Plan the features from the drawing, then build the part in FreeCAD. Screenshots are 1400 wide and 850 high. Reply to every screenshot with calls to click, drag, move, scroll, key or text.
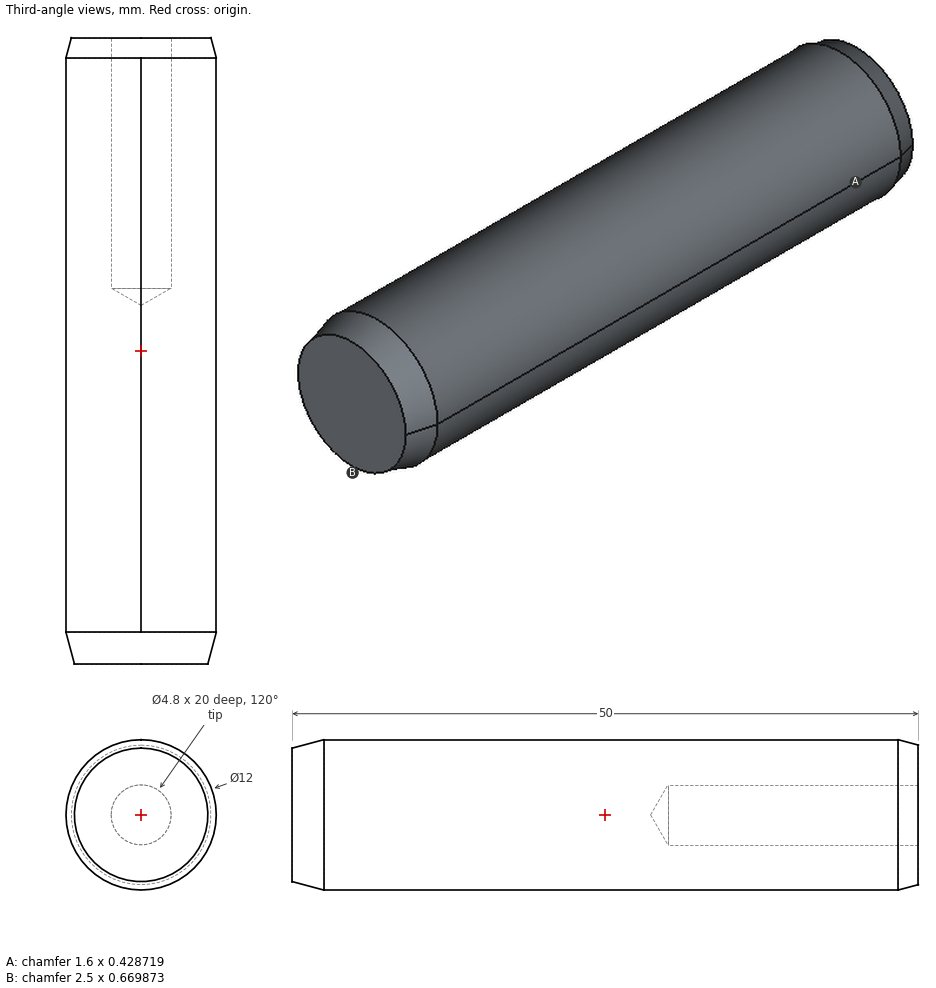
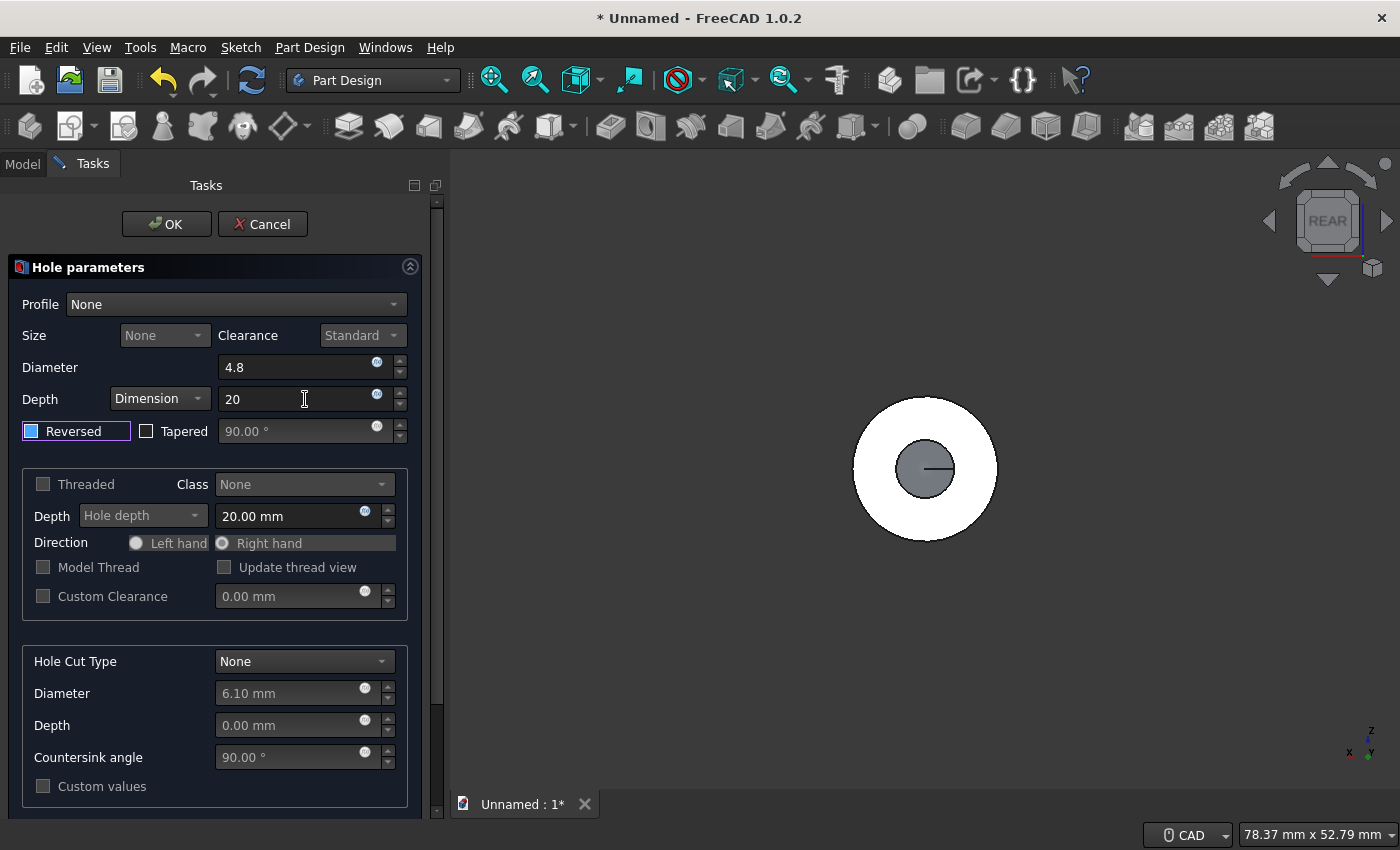
scroll(437, 506, down, 3)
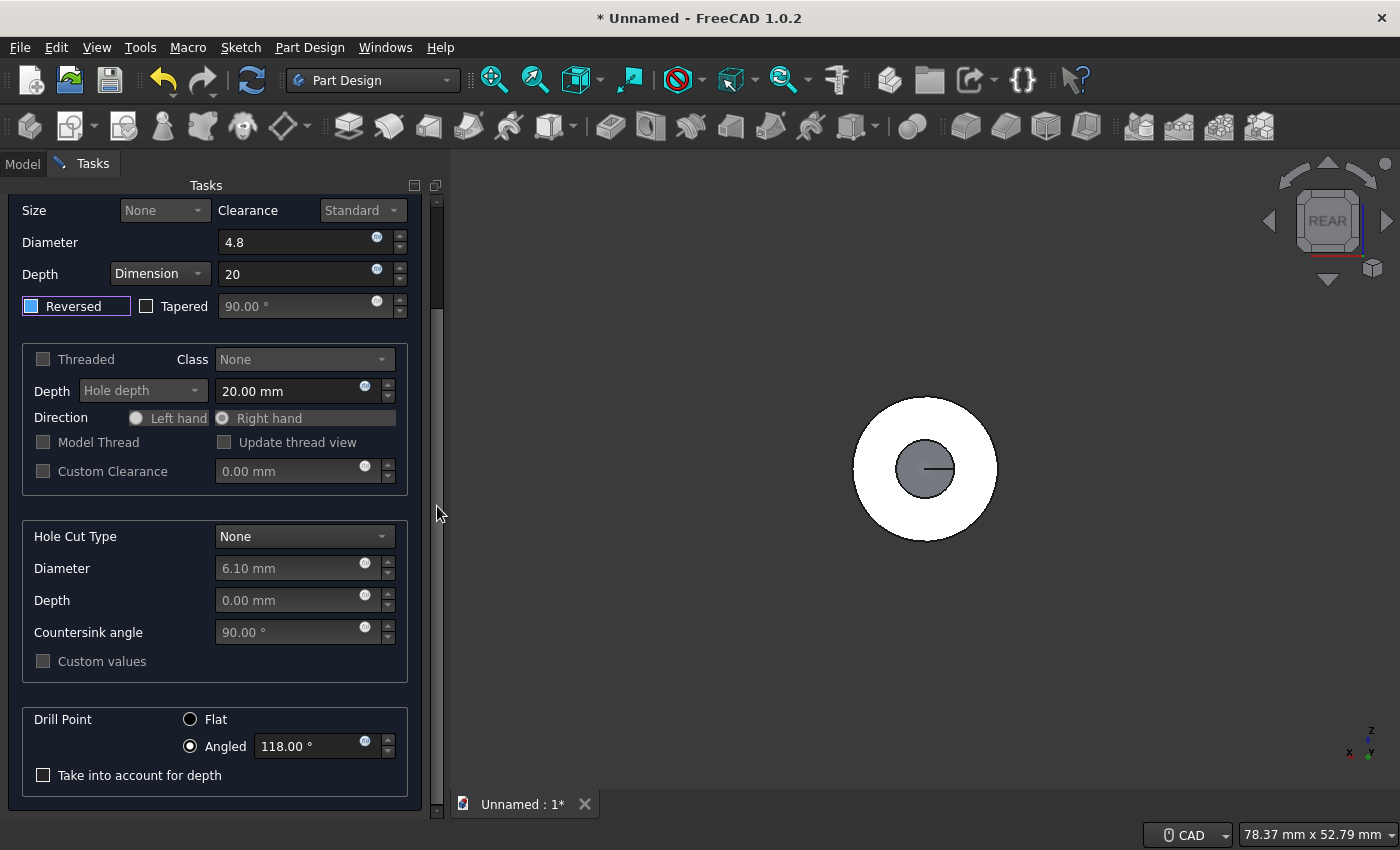
triple_click(317, 746)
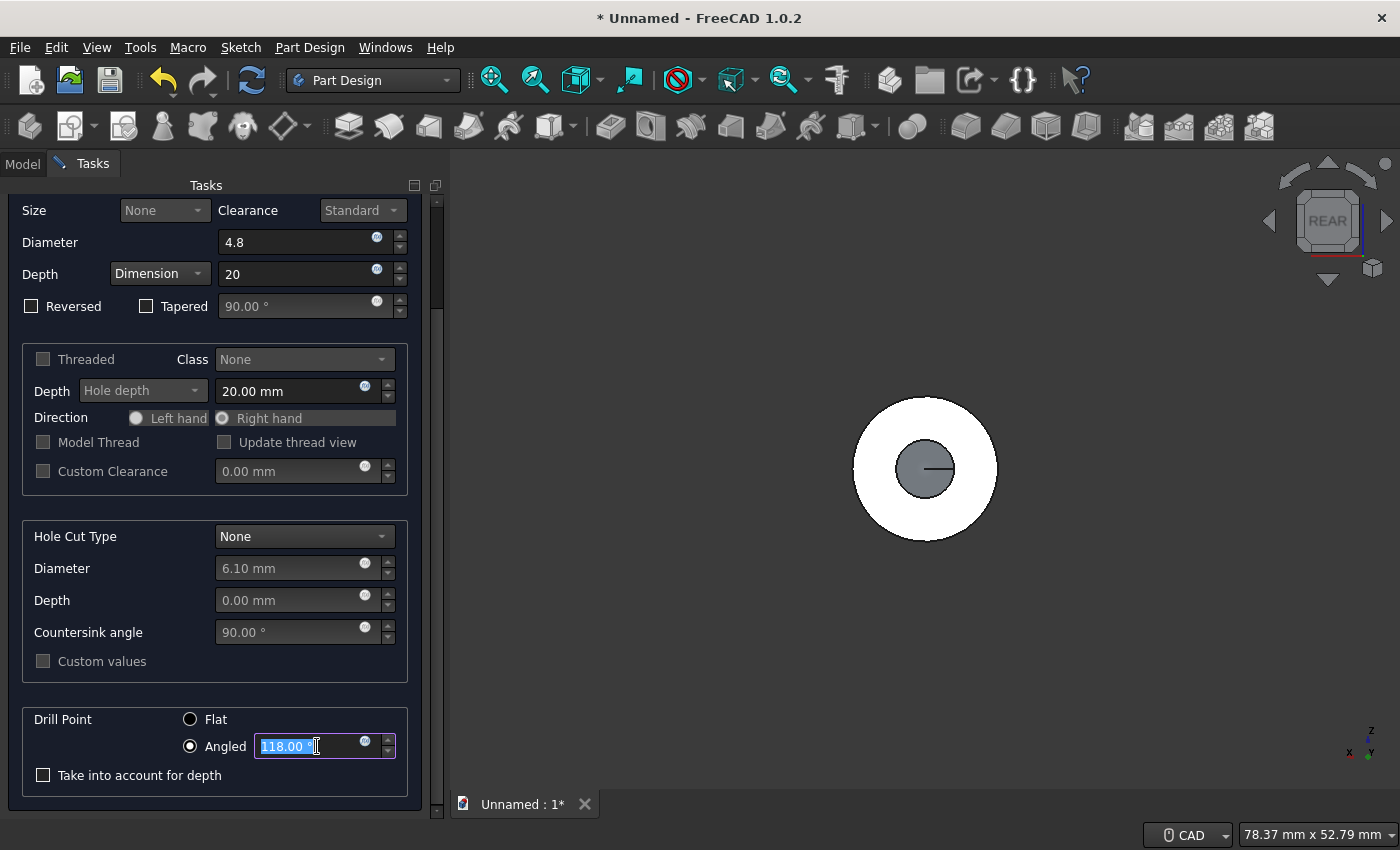
text(120)
key(Tab)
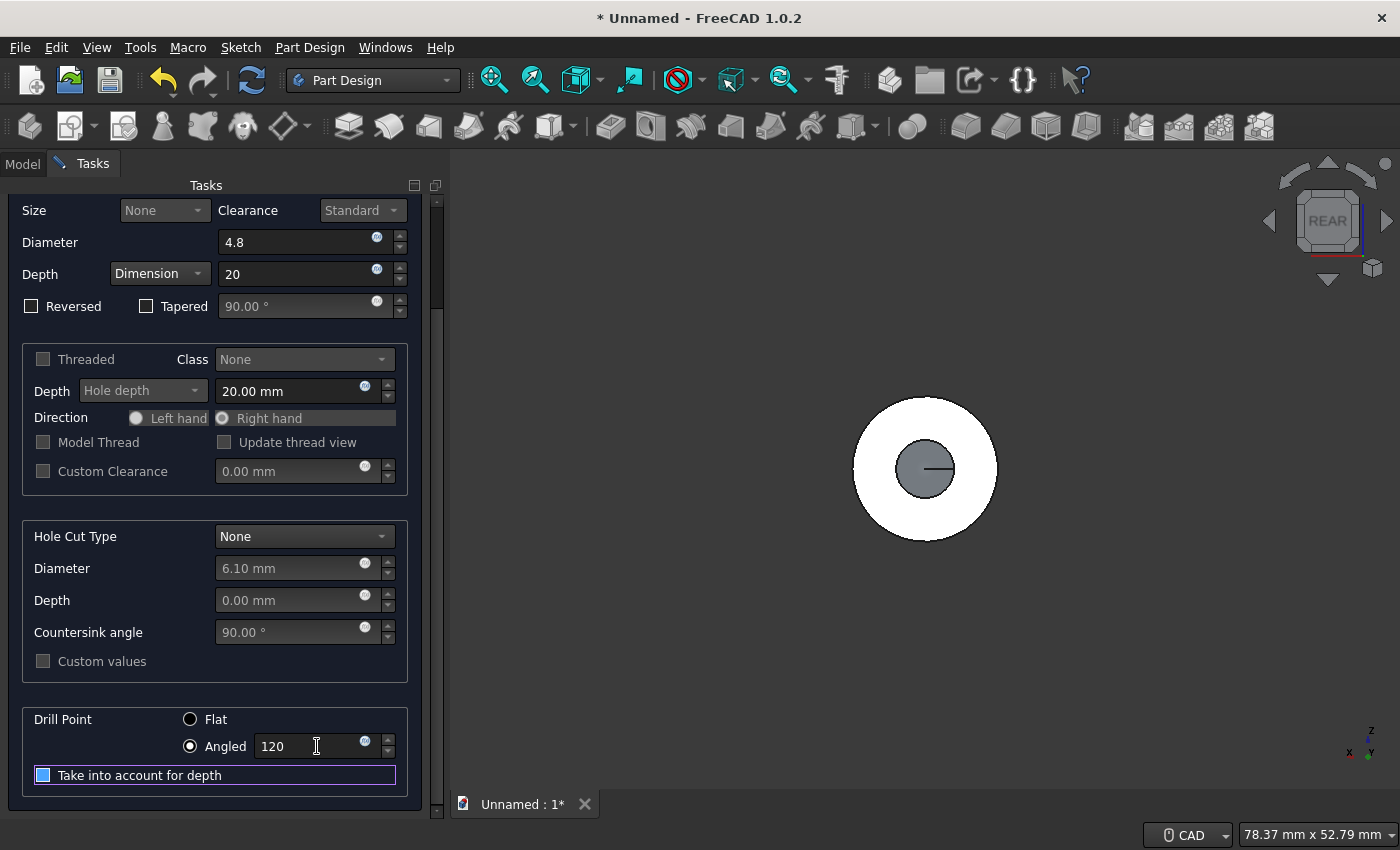
scroll(437, 506, up, 3)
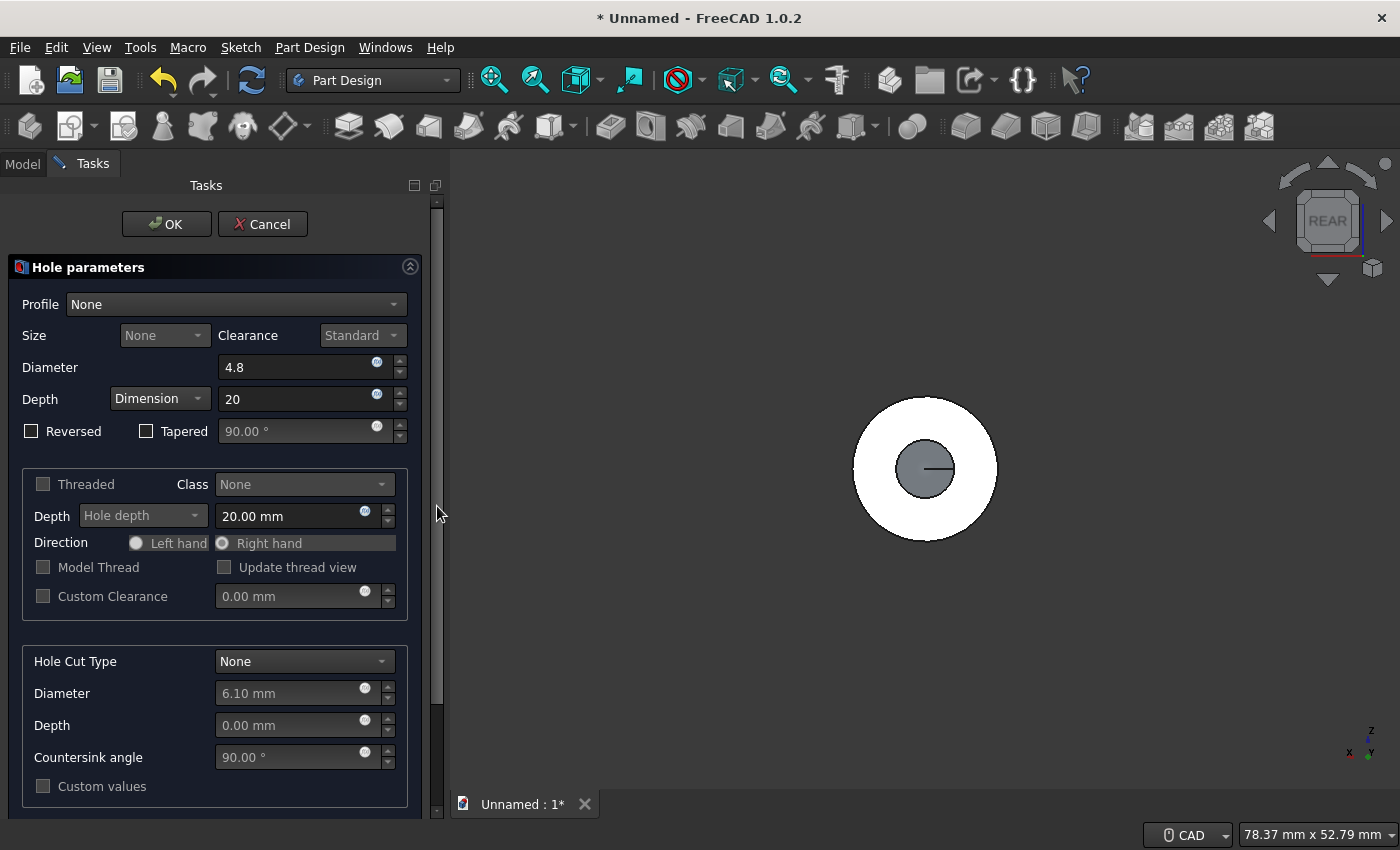
click(167, 224)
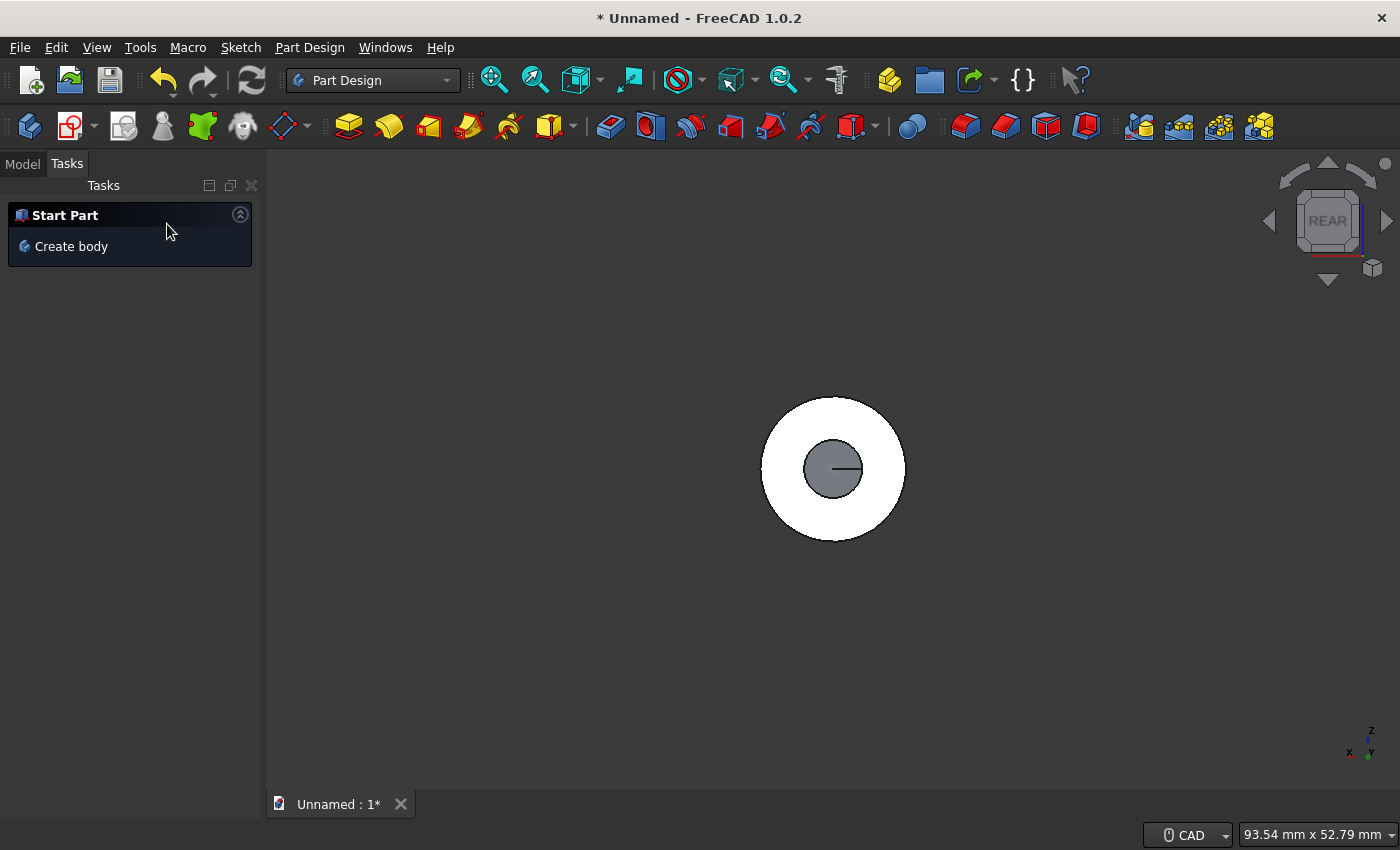
click(496, 80)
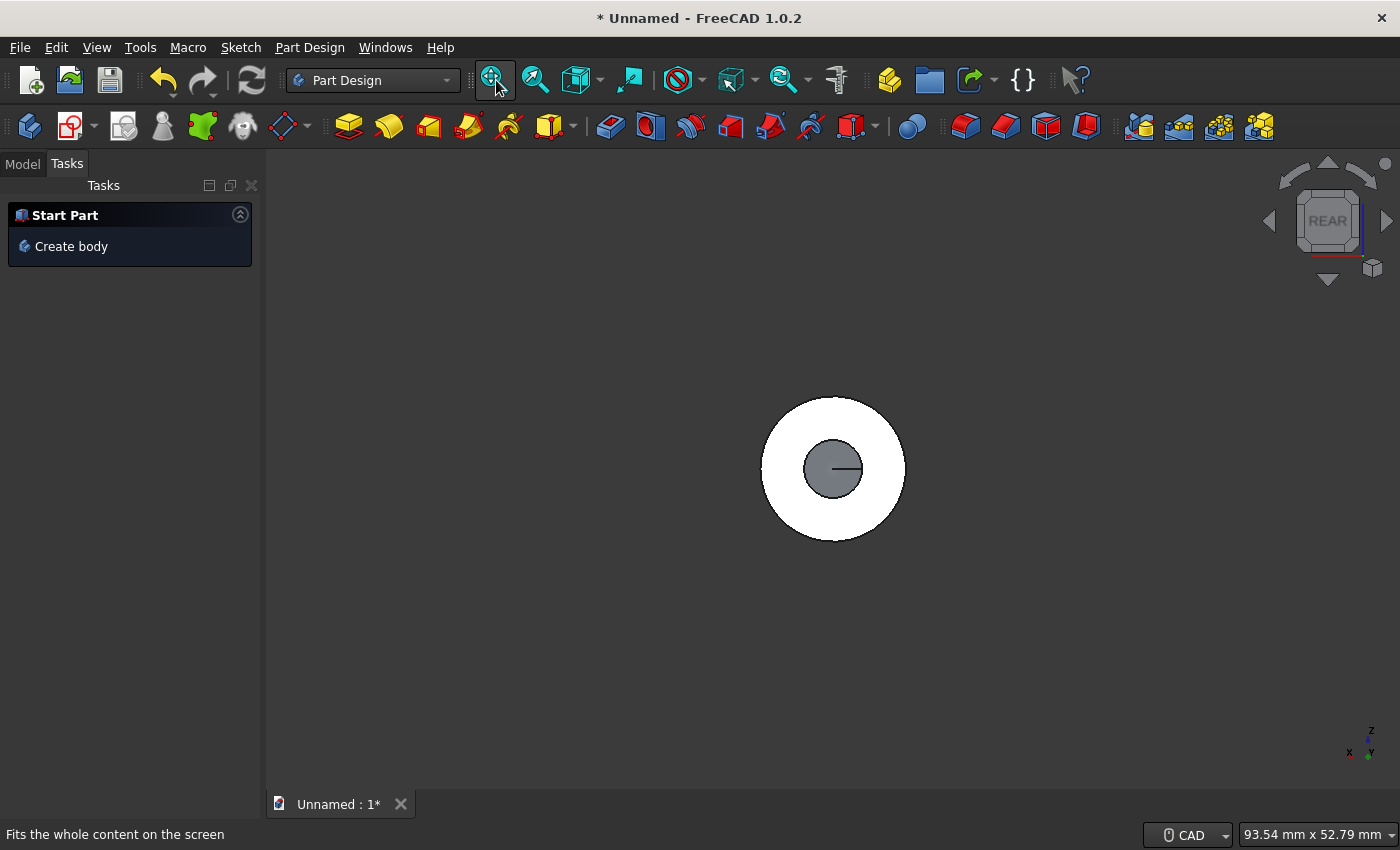
click(906, 468)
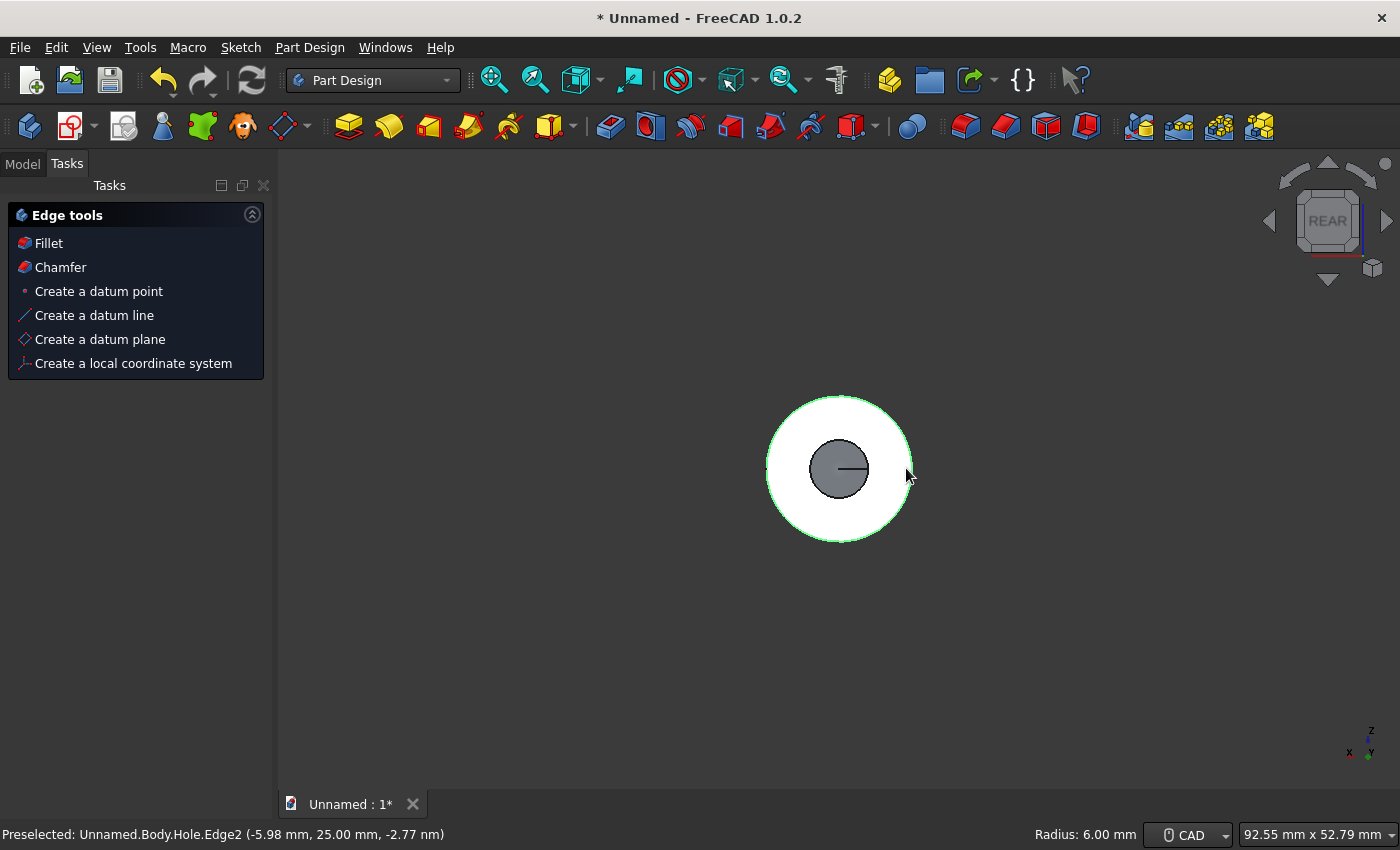
click(1006, 126)